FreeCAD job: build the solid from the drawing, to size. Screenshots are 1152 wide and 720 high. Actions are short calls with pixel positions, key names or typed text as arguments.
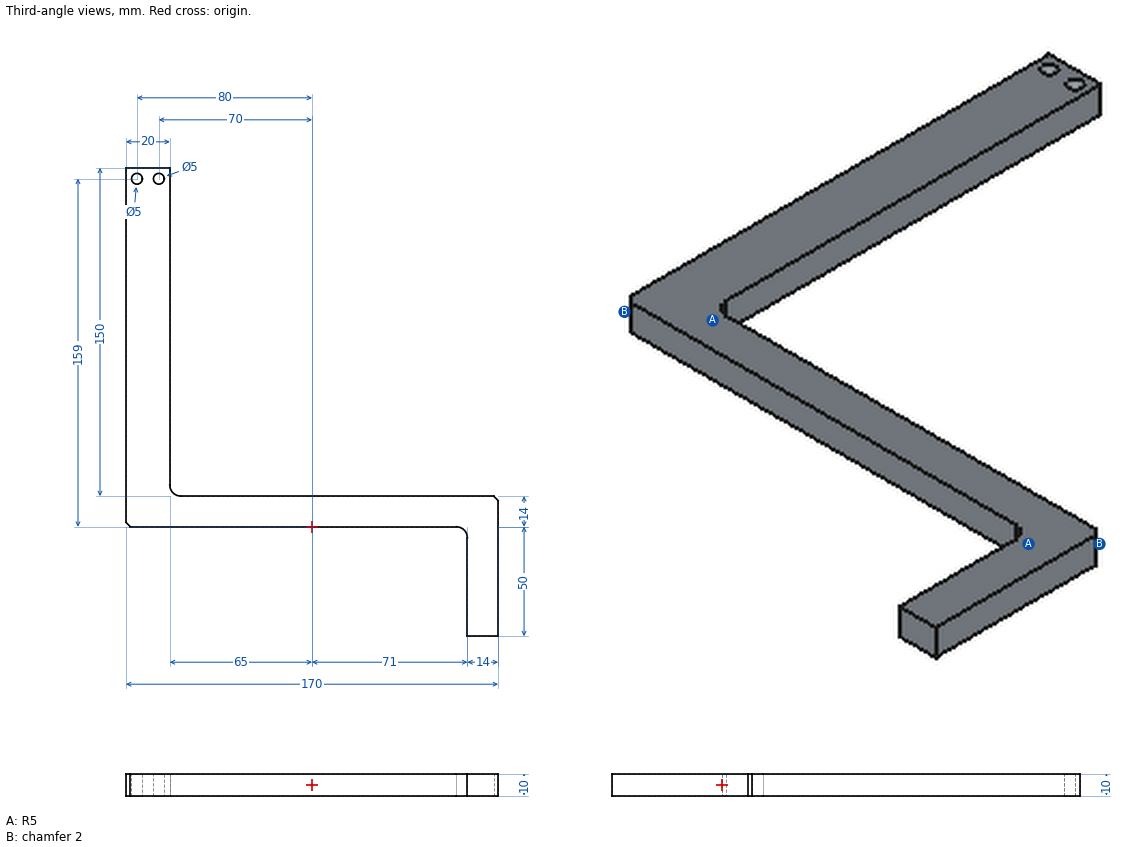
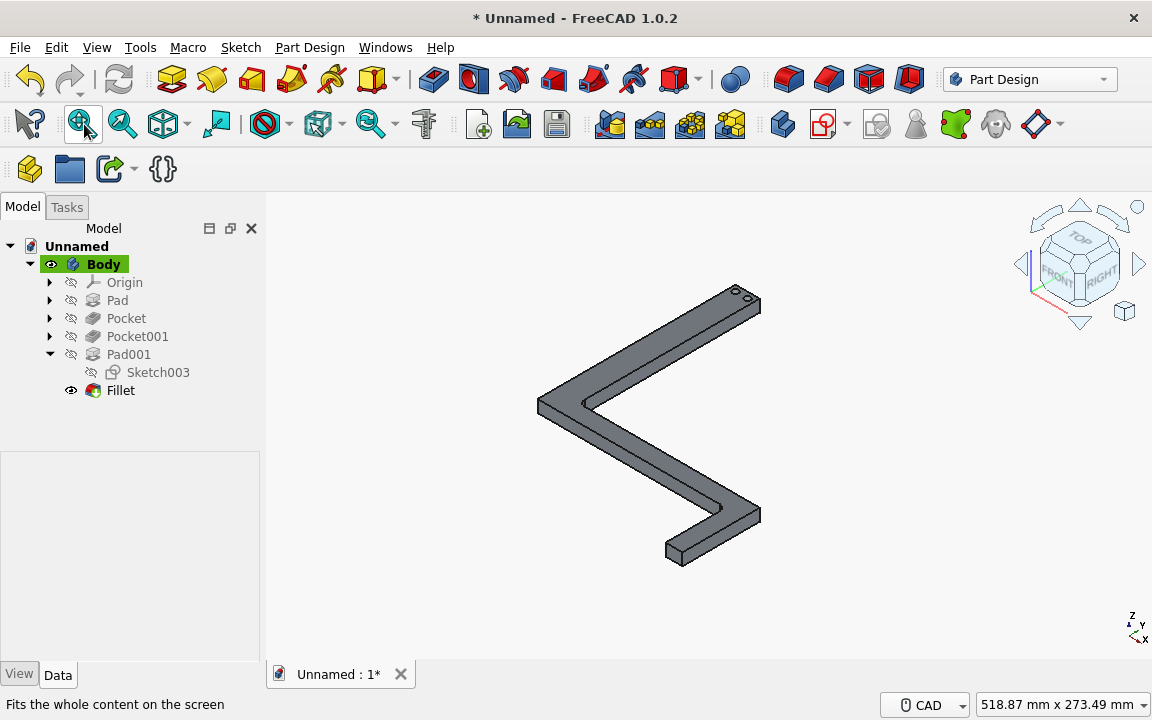
key(1)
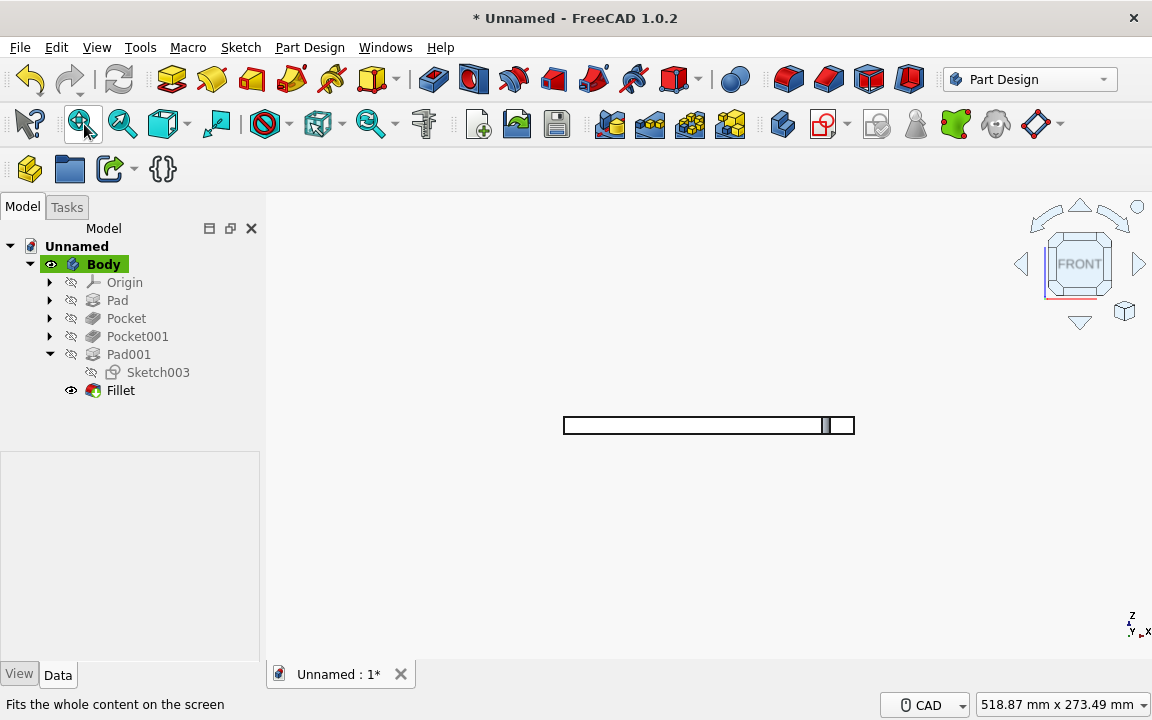
key(v)
key(f)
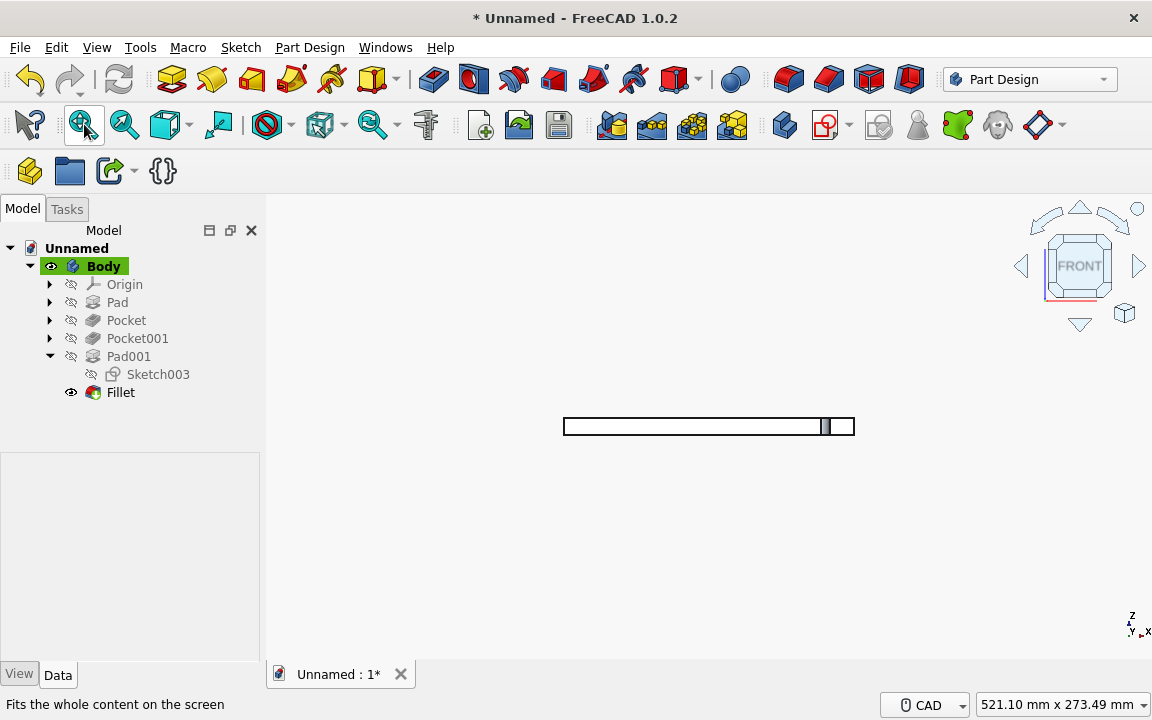
click(564, 426)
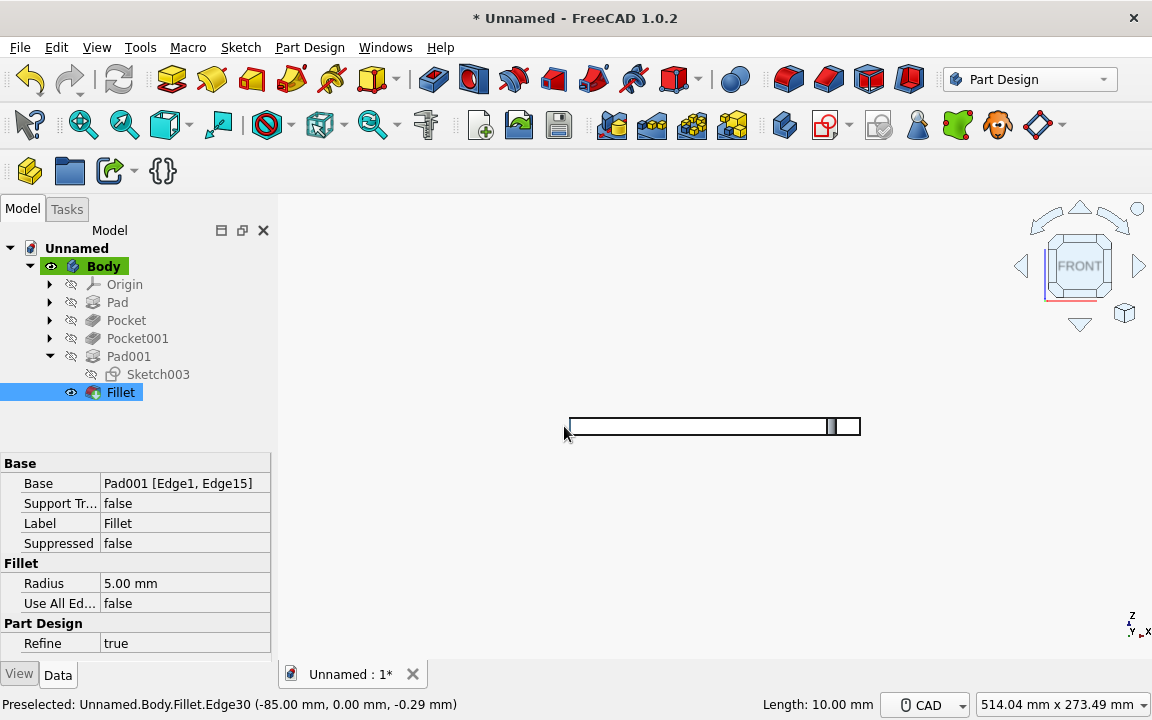
scroll(860, 426, up, 5)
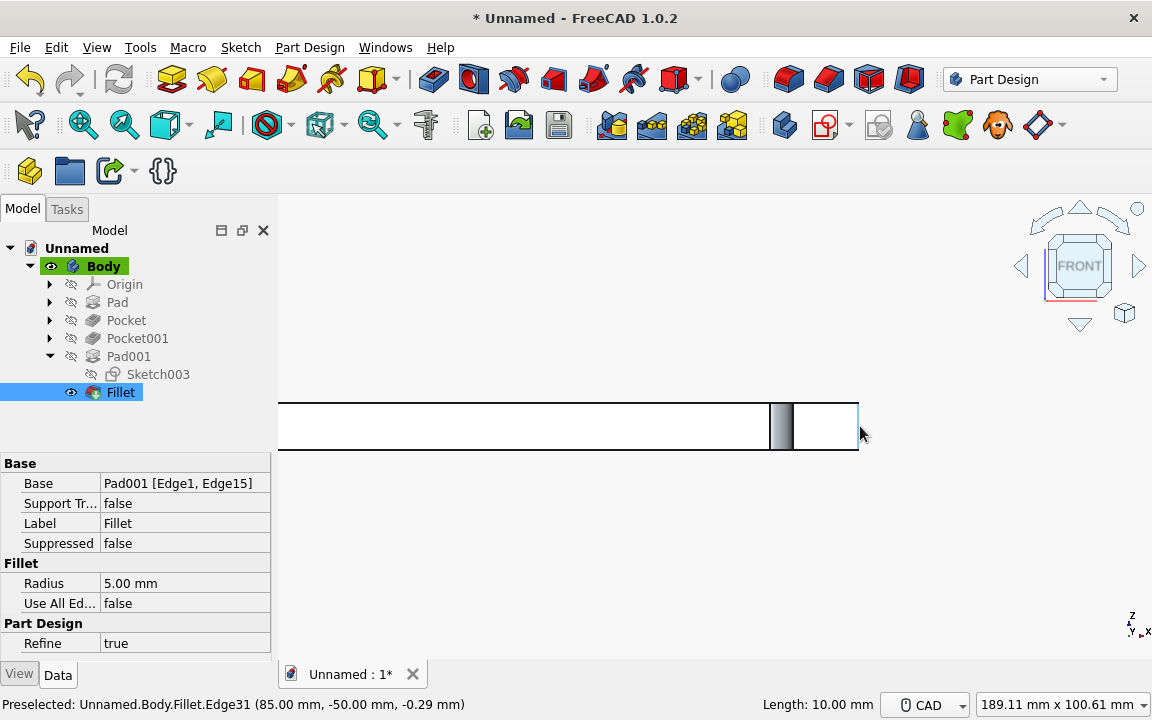
click(84, 126)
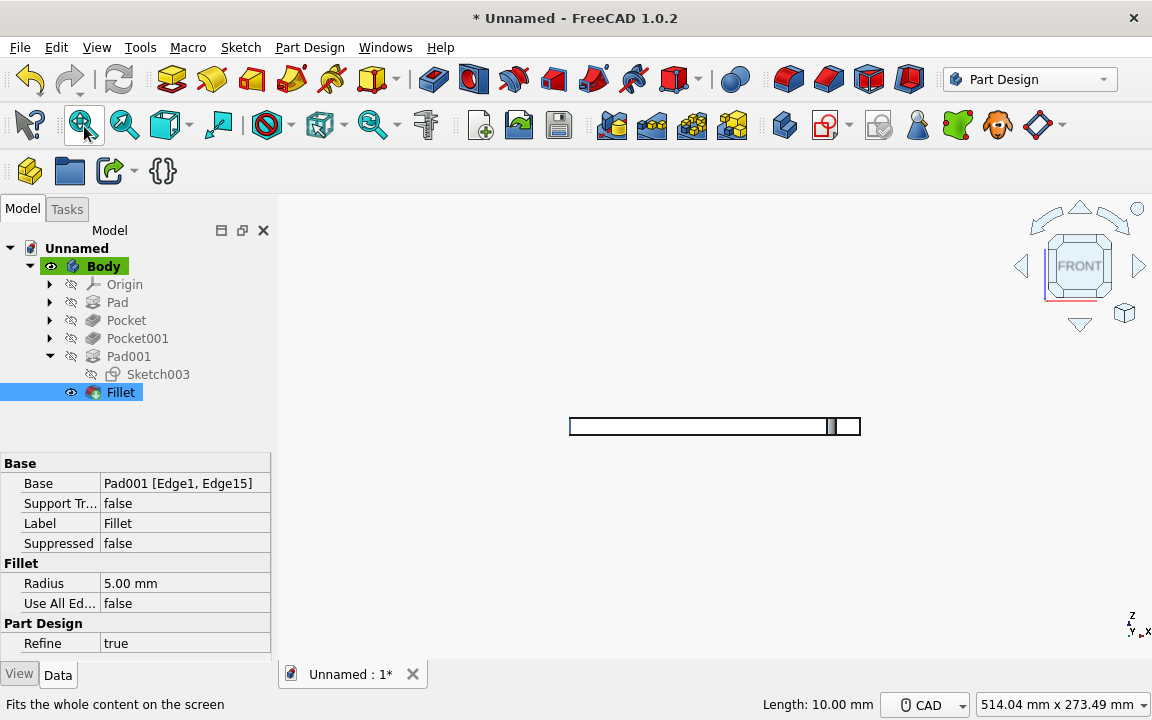
key(3)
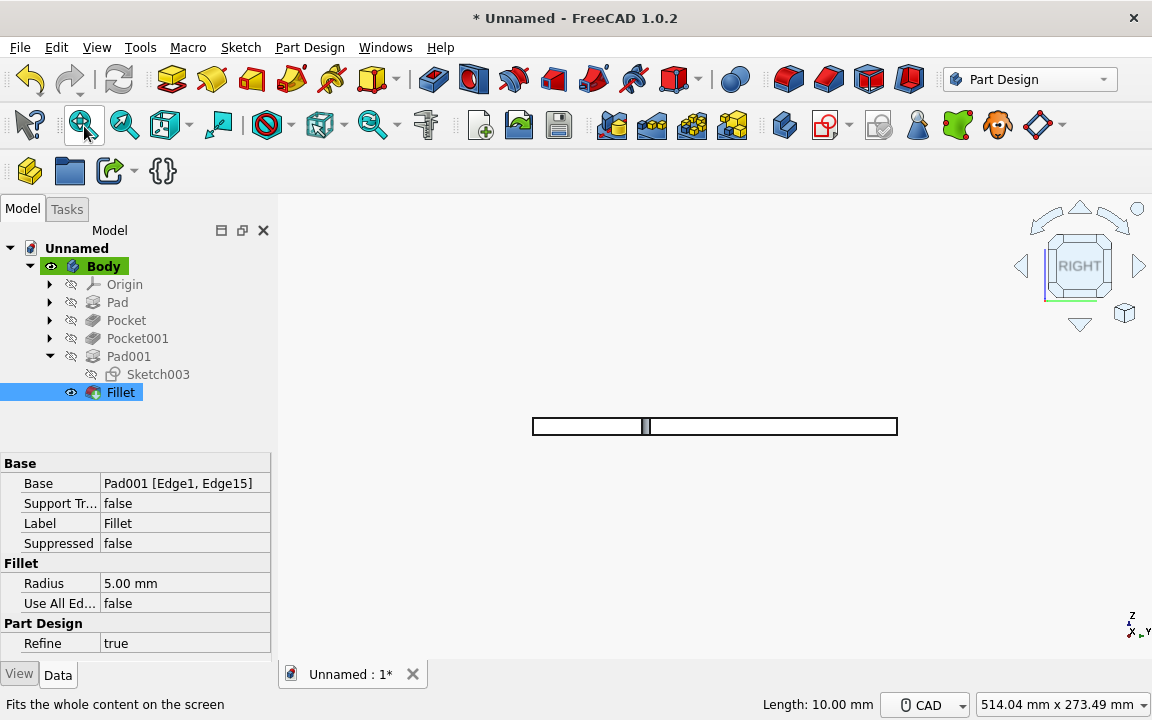
key(v)
key(f)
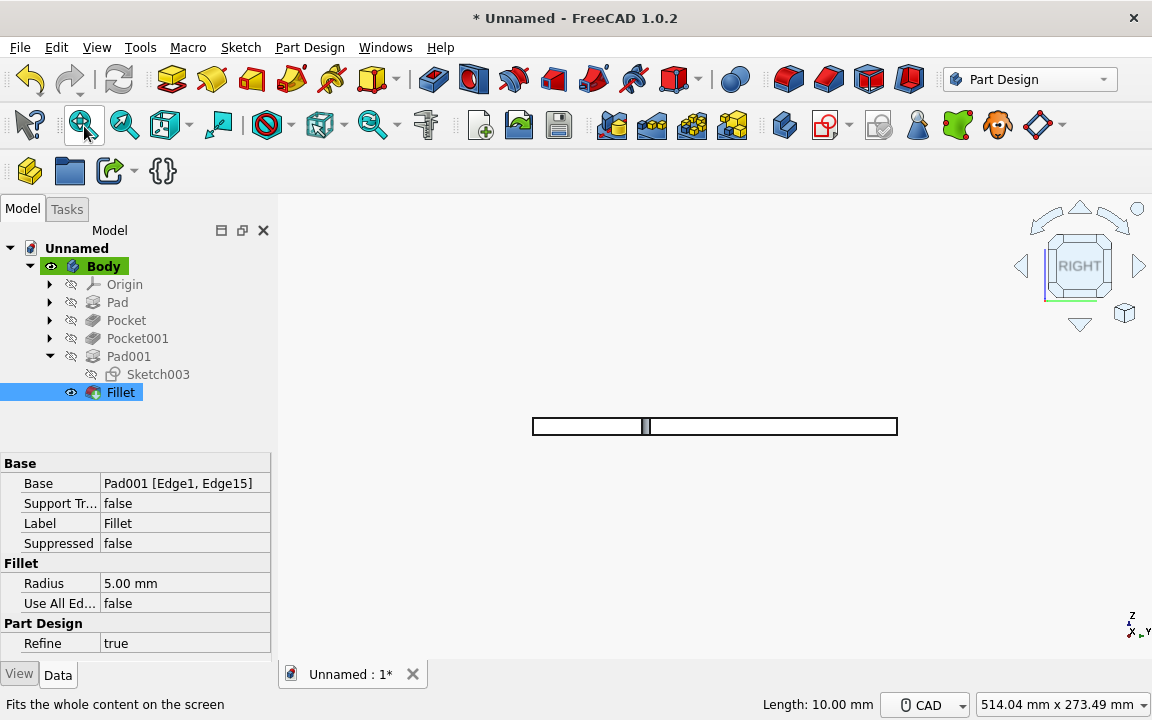
click(642, 425, ctrl)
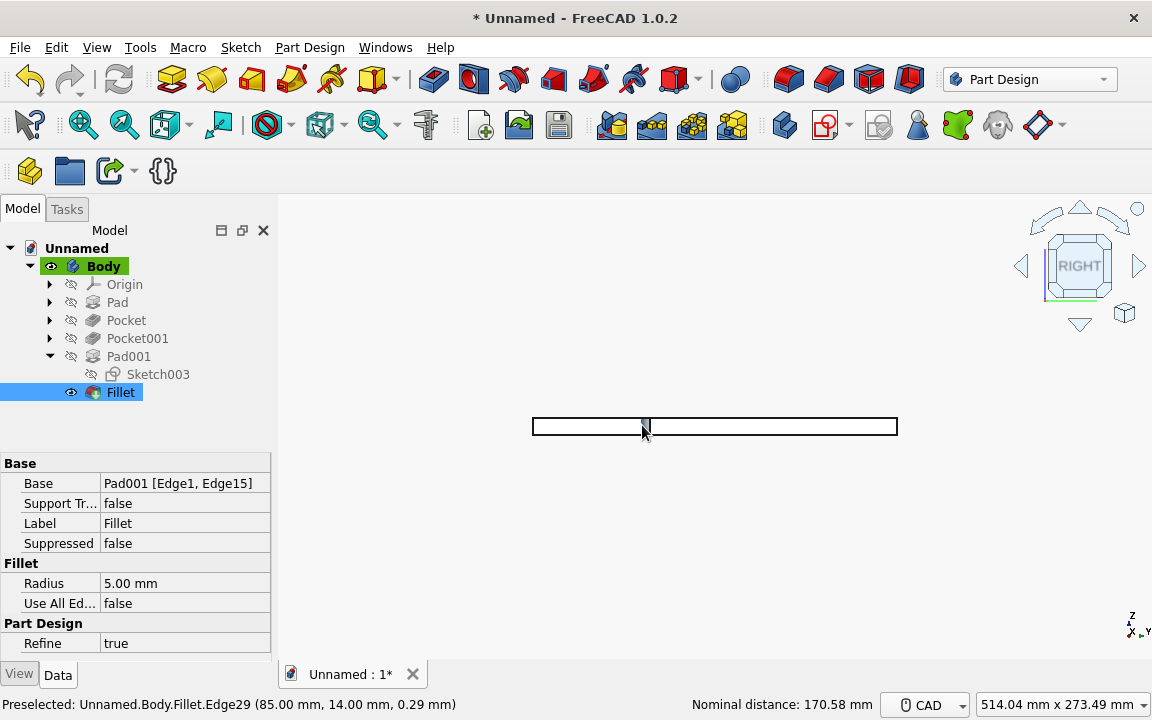
click(830, 80)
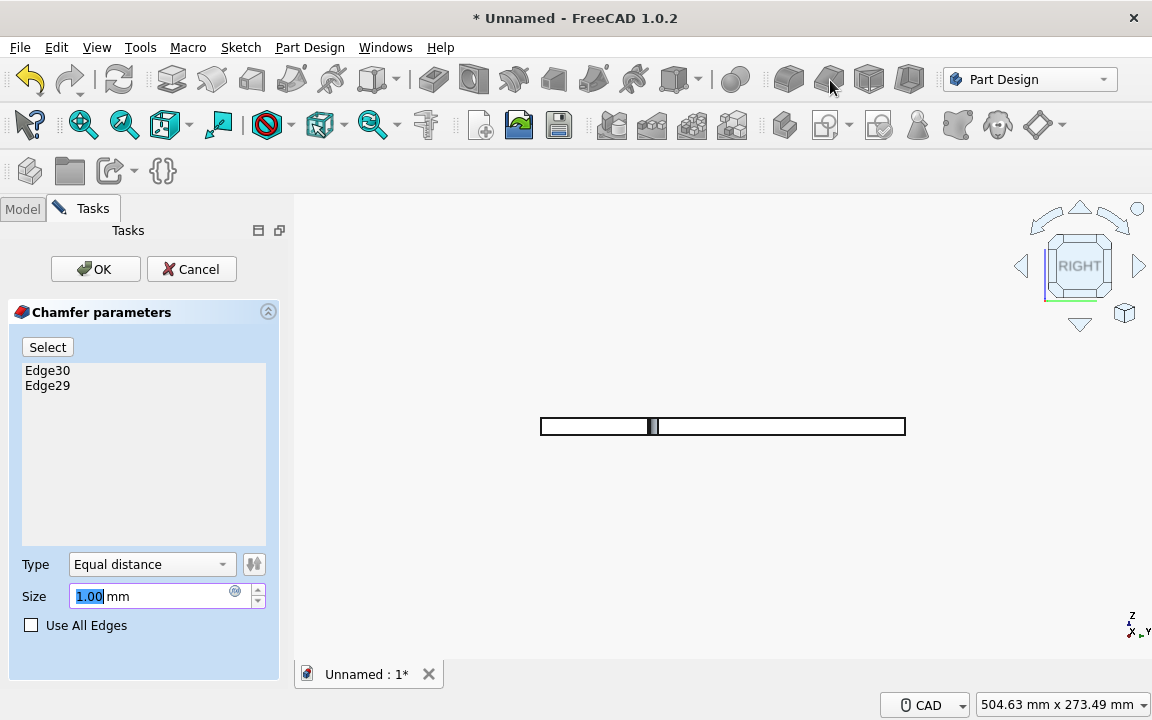
text(2)
key(Tab)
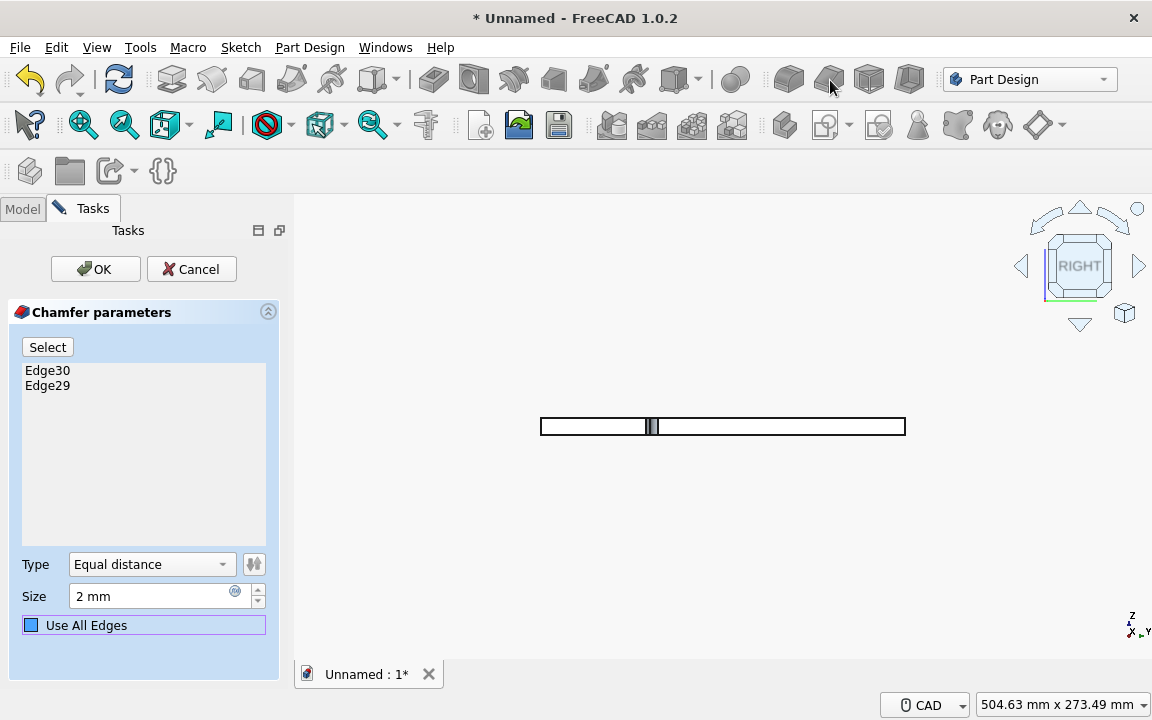
click(96, 269)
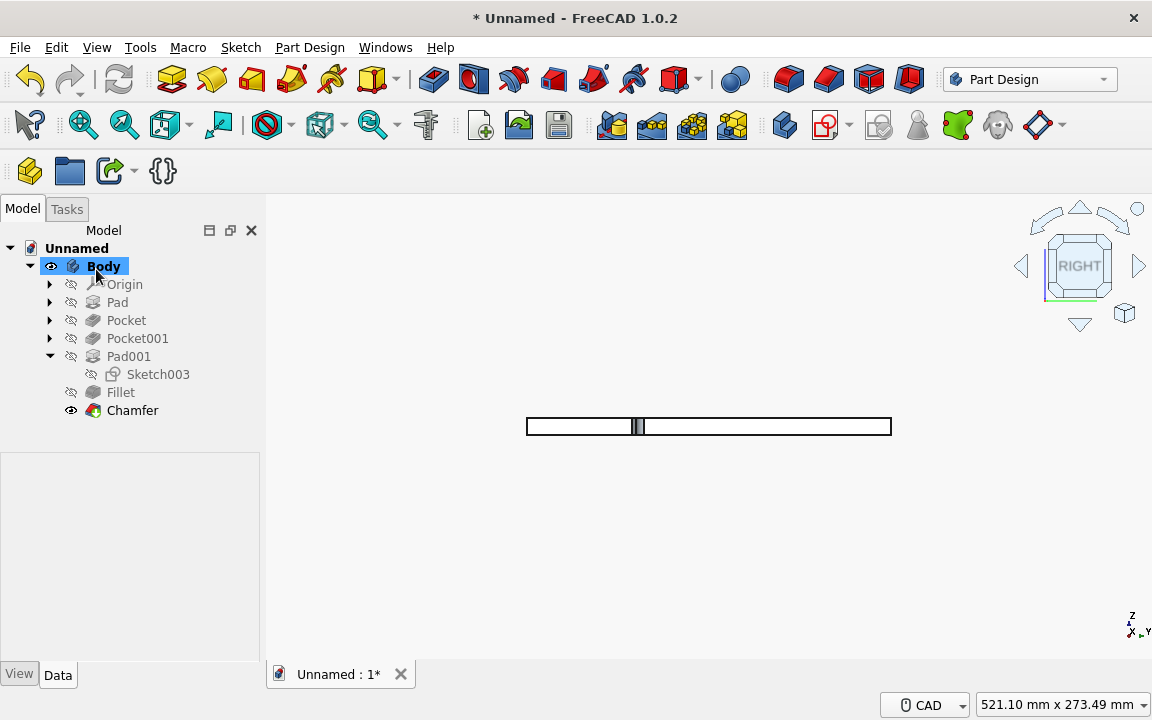
key(0)